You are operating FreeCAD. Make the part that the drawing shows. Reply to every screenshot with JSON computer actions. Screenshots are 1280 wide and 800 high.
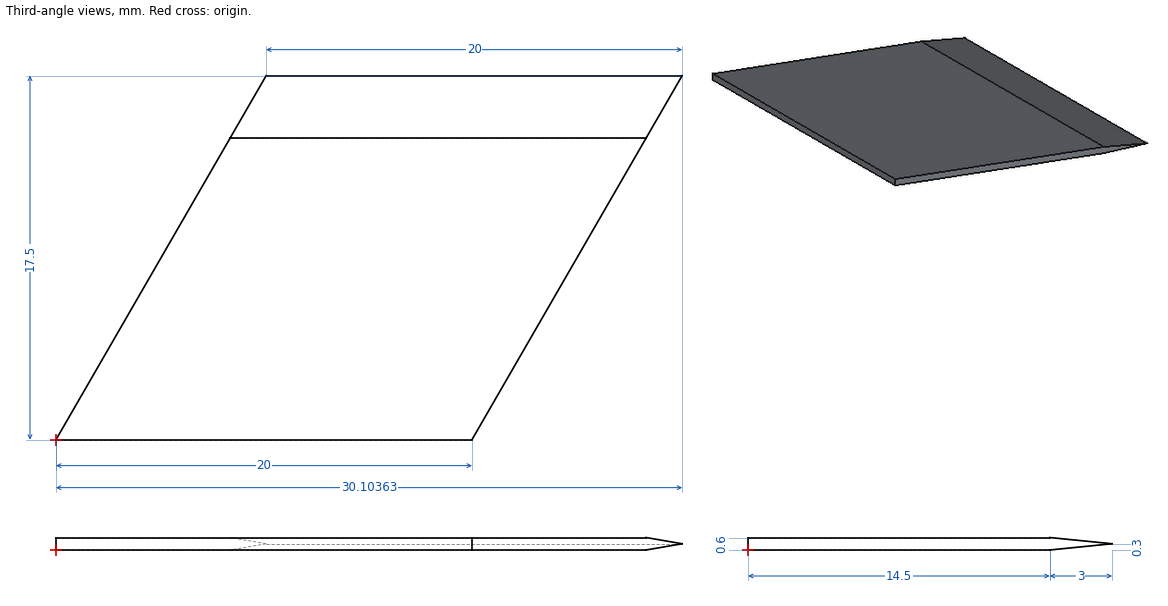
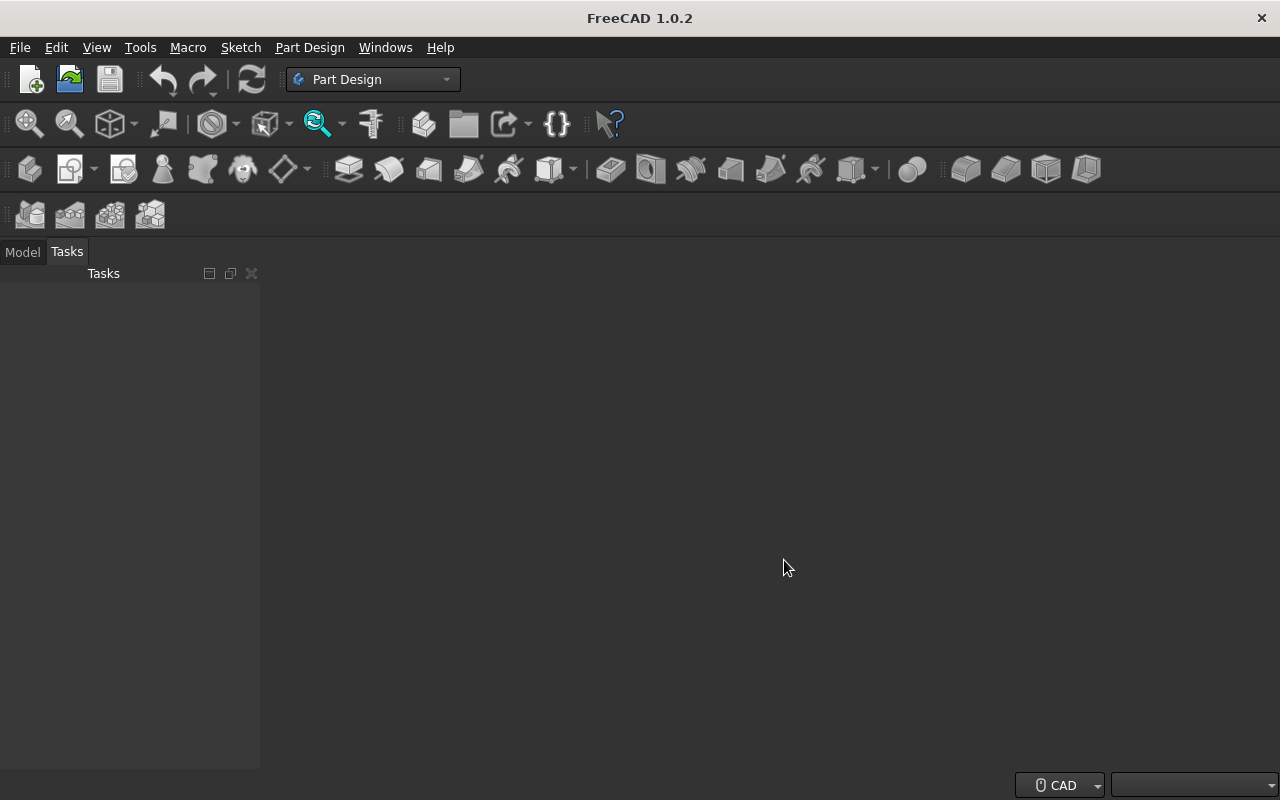
{"action": "left_click", "coordinate": [30, 80]}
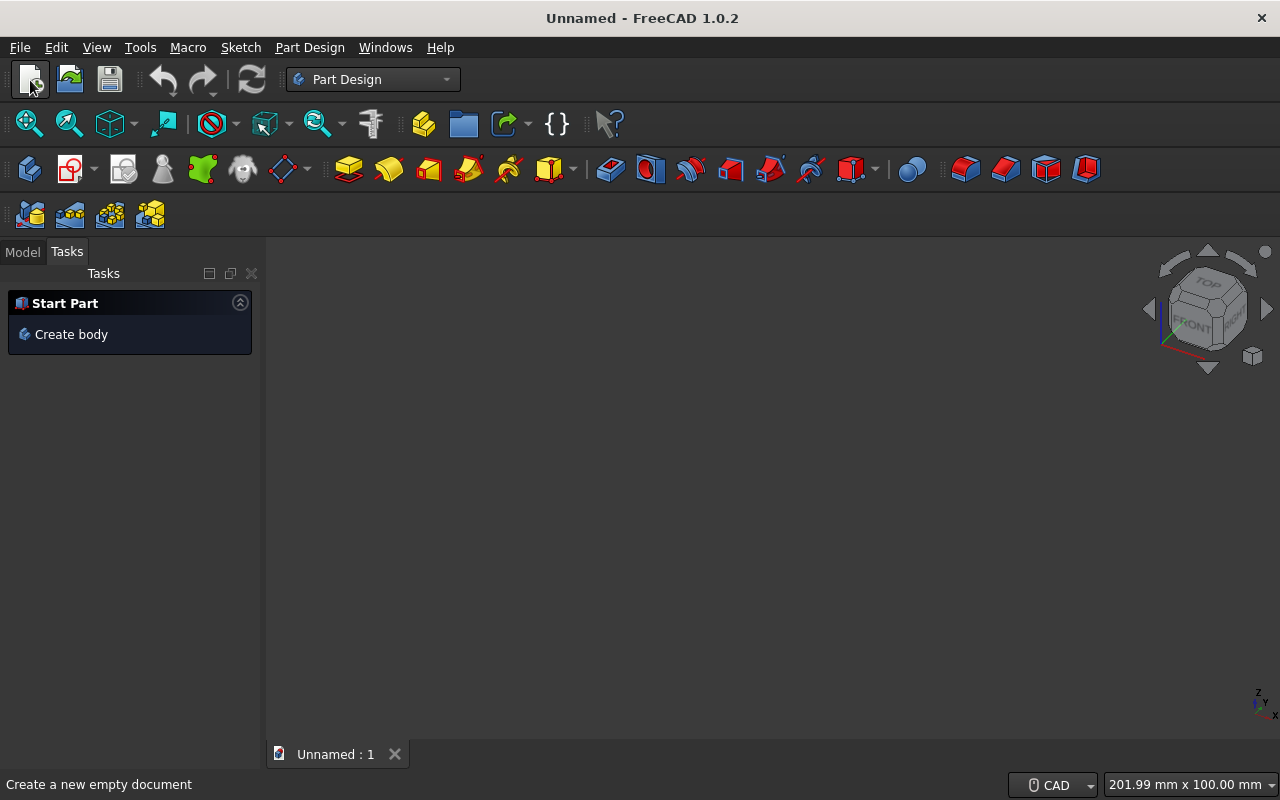
{"action": "left_click", "coordinate": [70, 170]}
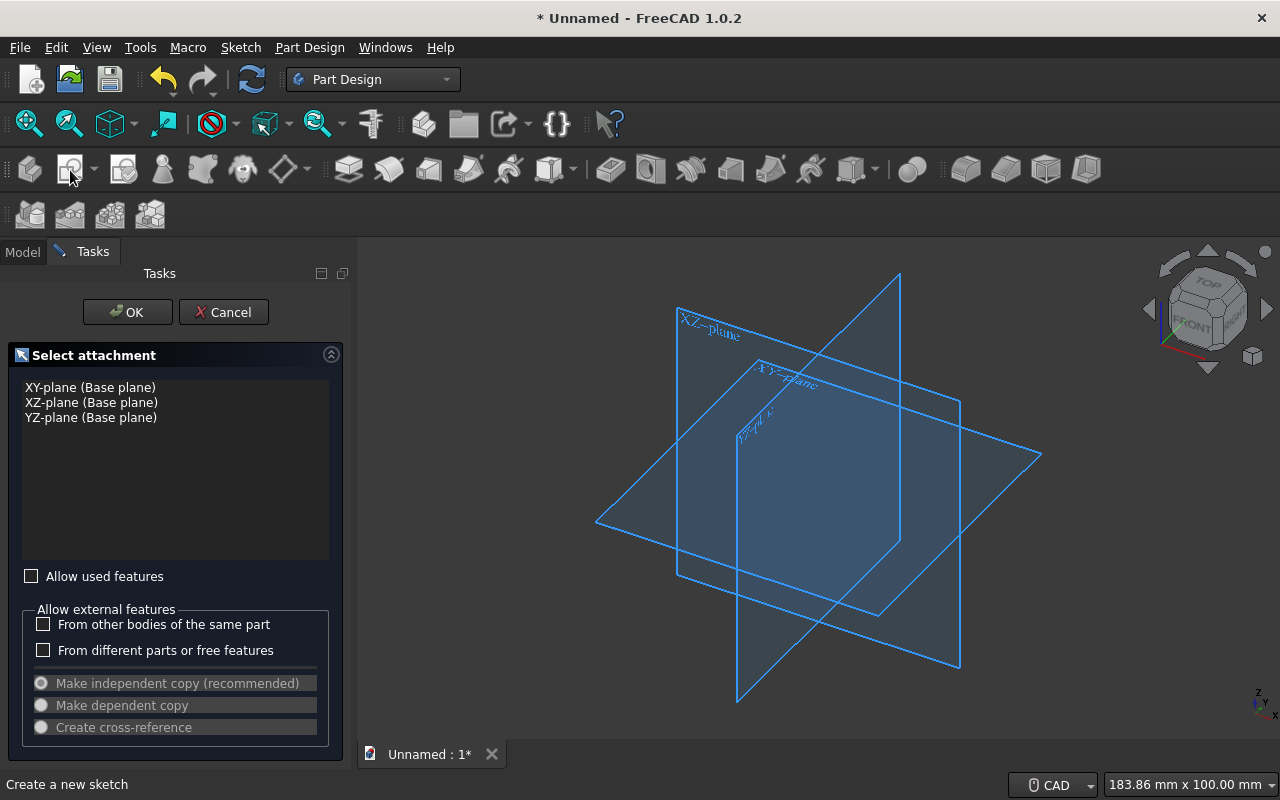
{"action": "left_click", "coordinate": [82, 388]}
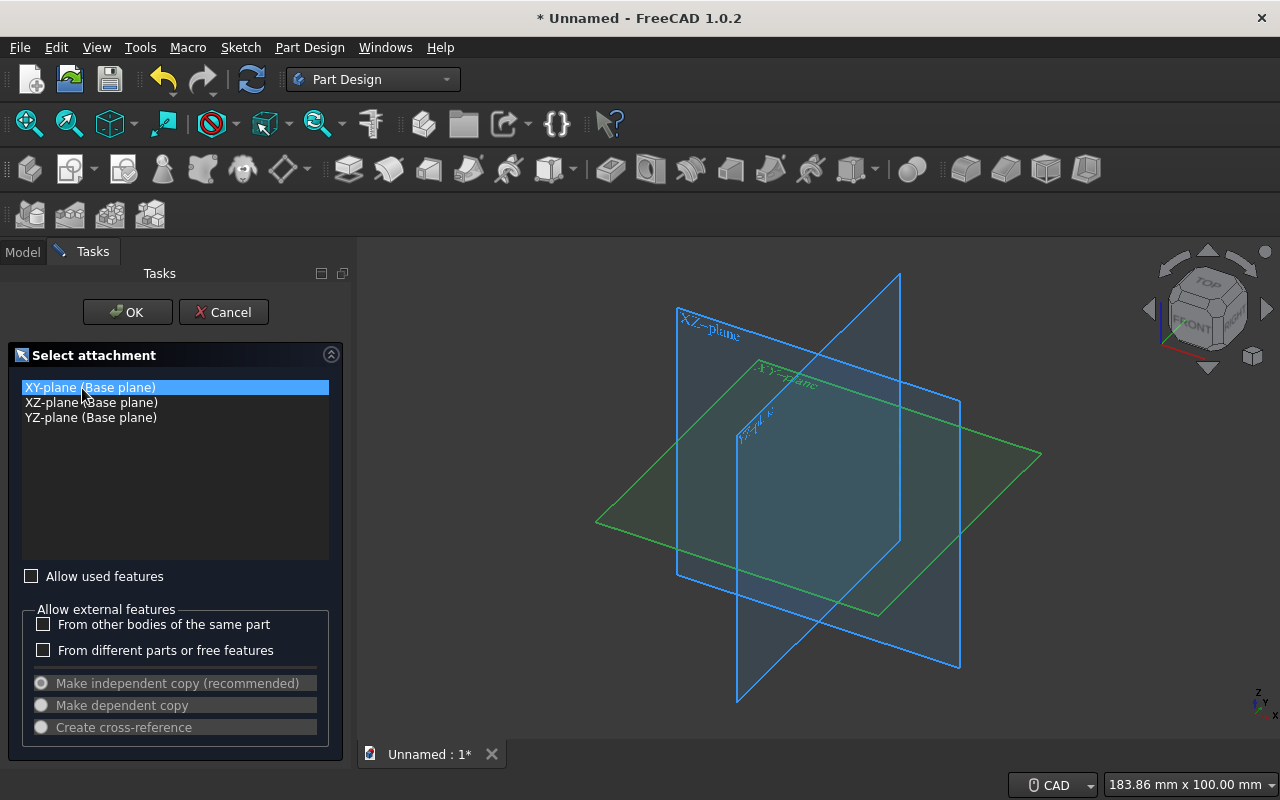
{"action": "left_click", "coordinate": [128, 312]}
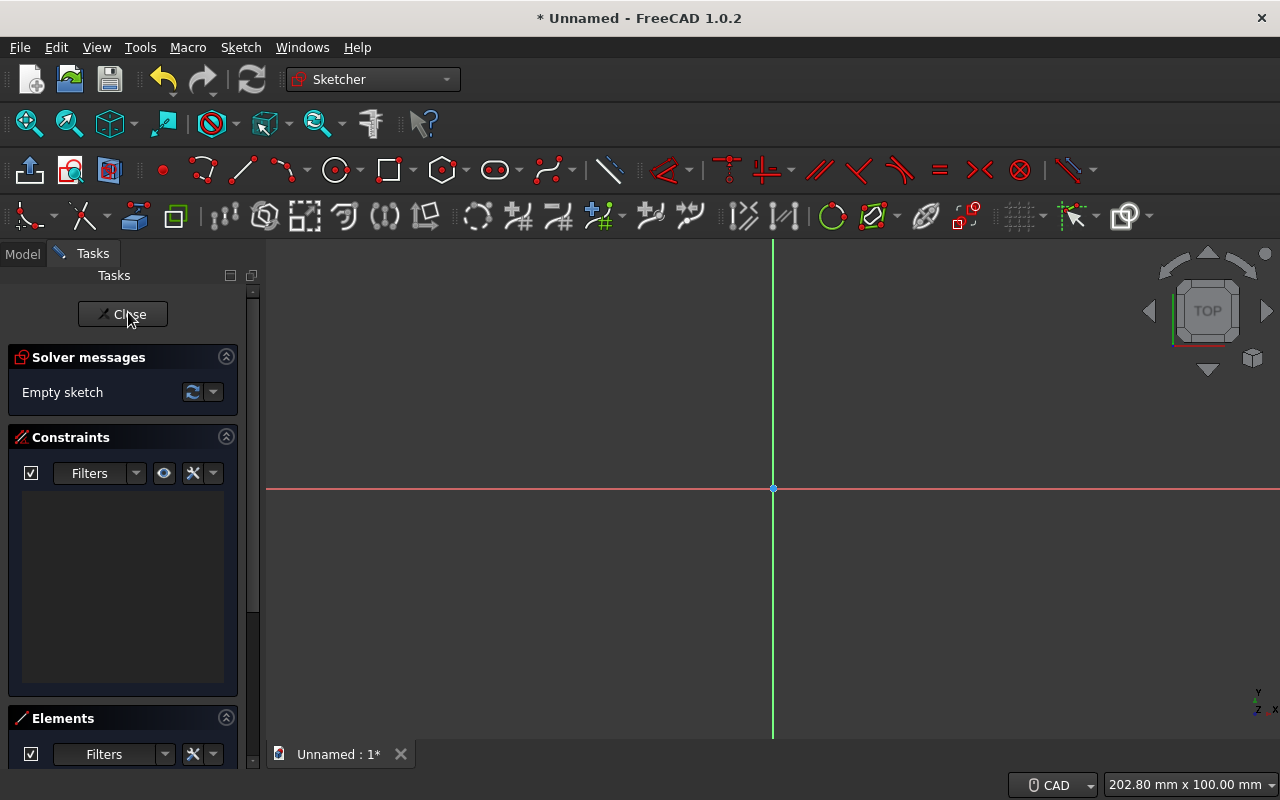
{"action": "scroll", "coordinate": [910, 426], "scroll_direction": "up", "scroll_amount": 6}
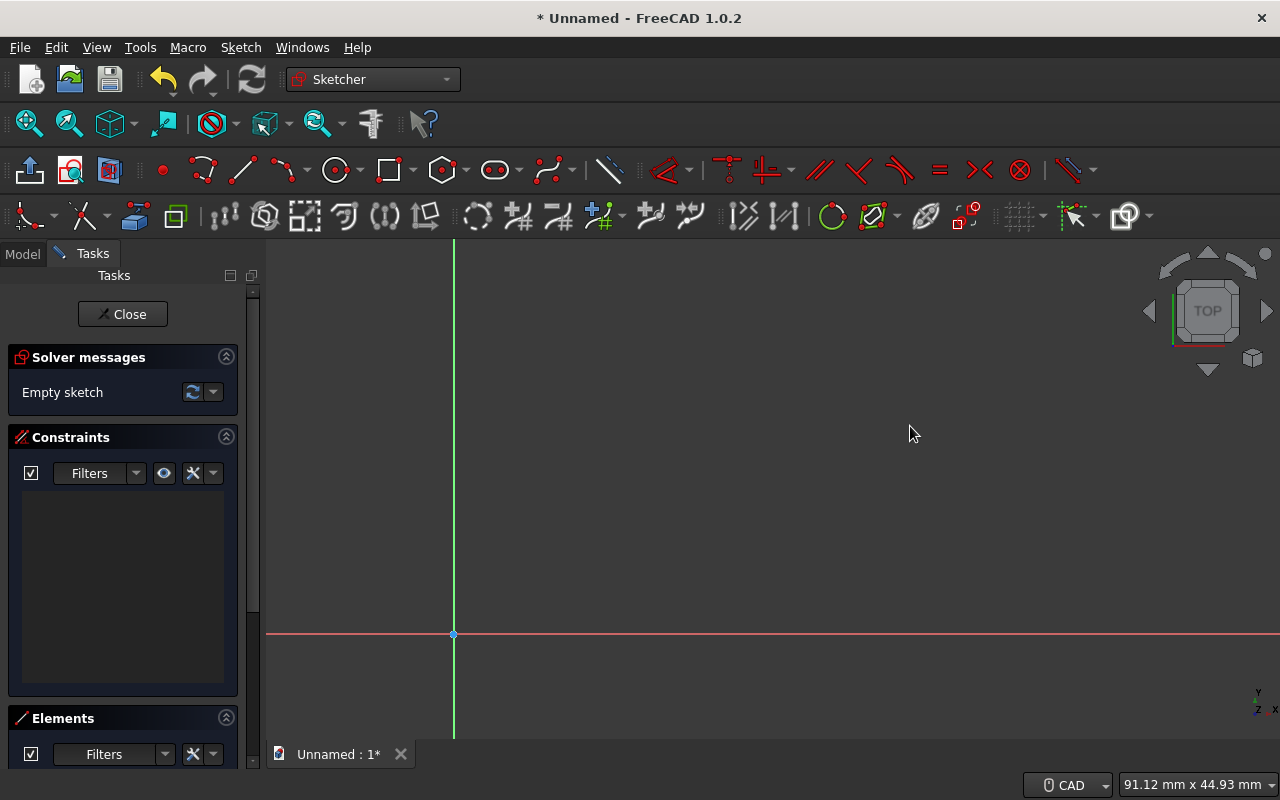
{"action": "left_click", "coordinate": [204, 170]}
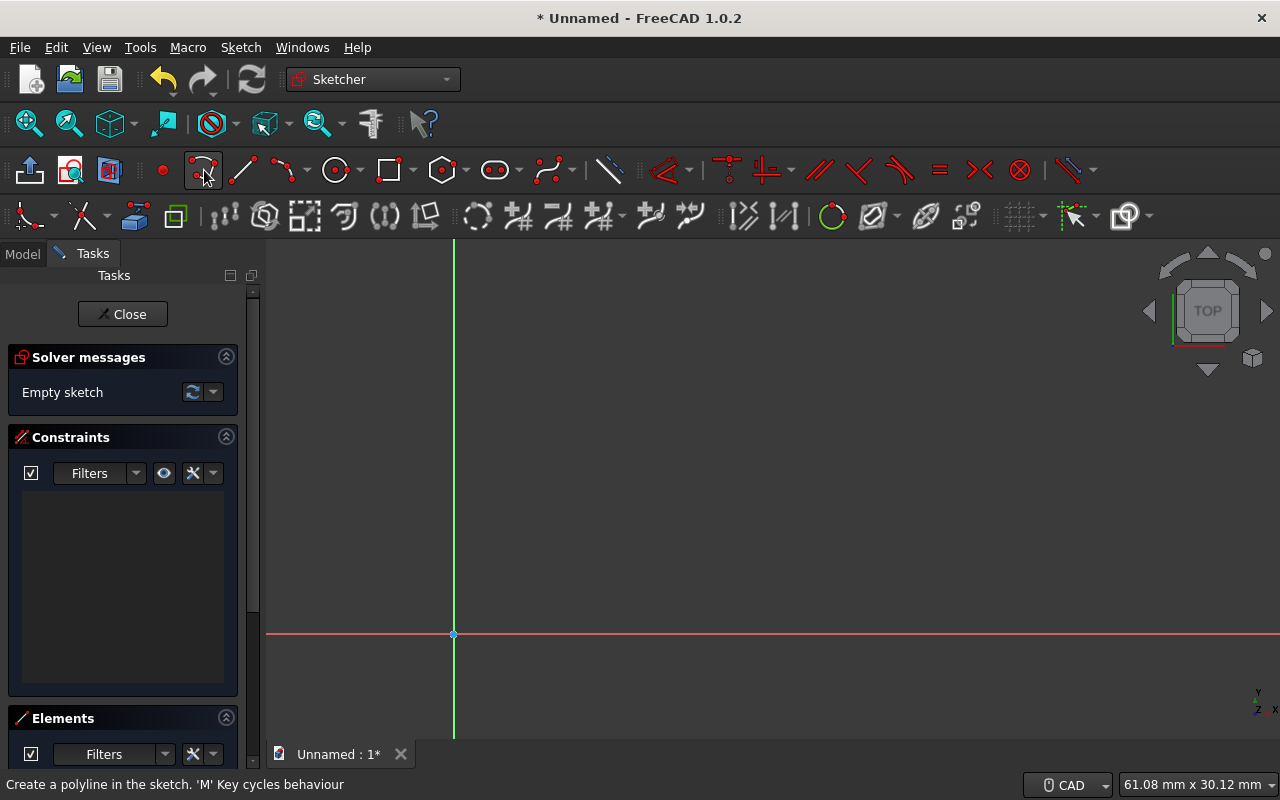
{"action": "left_click", "coordinate": [454, 634]}
{"action": "left_click", "coordinate": [786, 625]}
{"action": "left_click", "coordinate": [953, 344]}
{"action": "left_click", "coordinate": [621, 344]}
{"action": "left_click", "coordinate": [454, 634]}
{"action": "key", "text": "Escape"}
{"action": "key", "text": "Escape"}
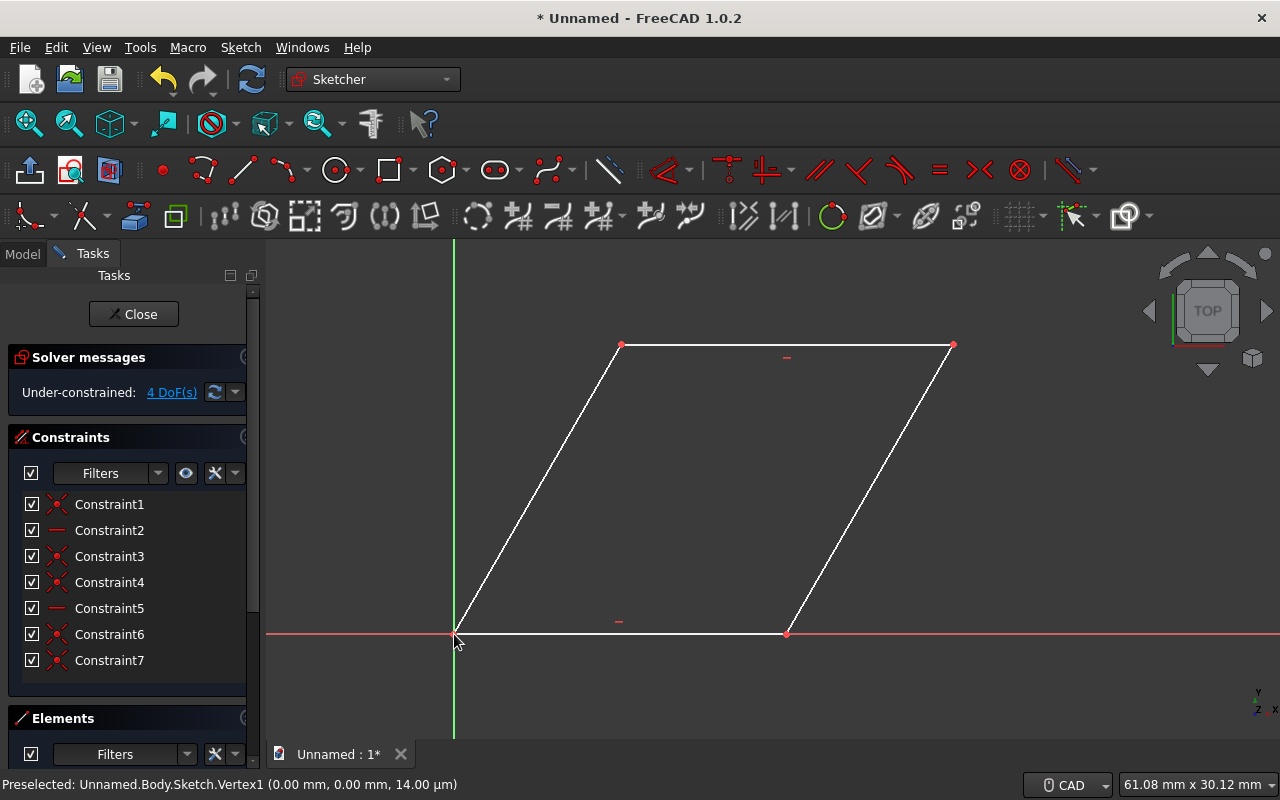
{"action": "left_click", "coordinate": [553, 634]}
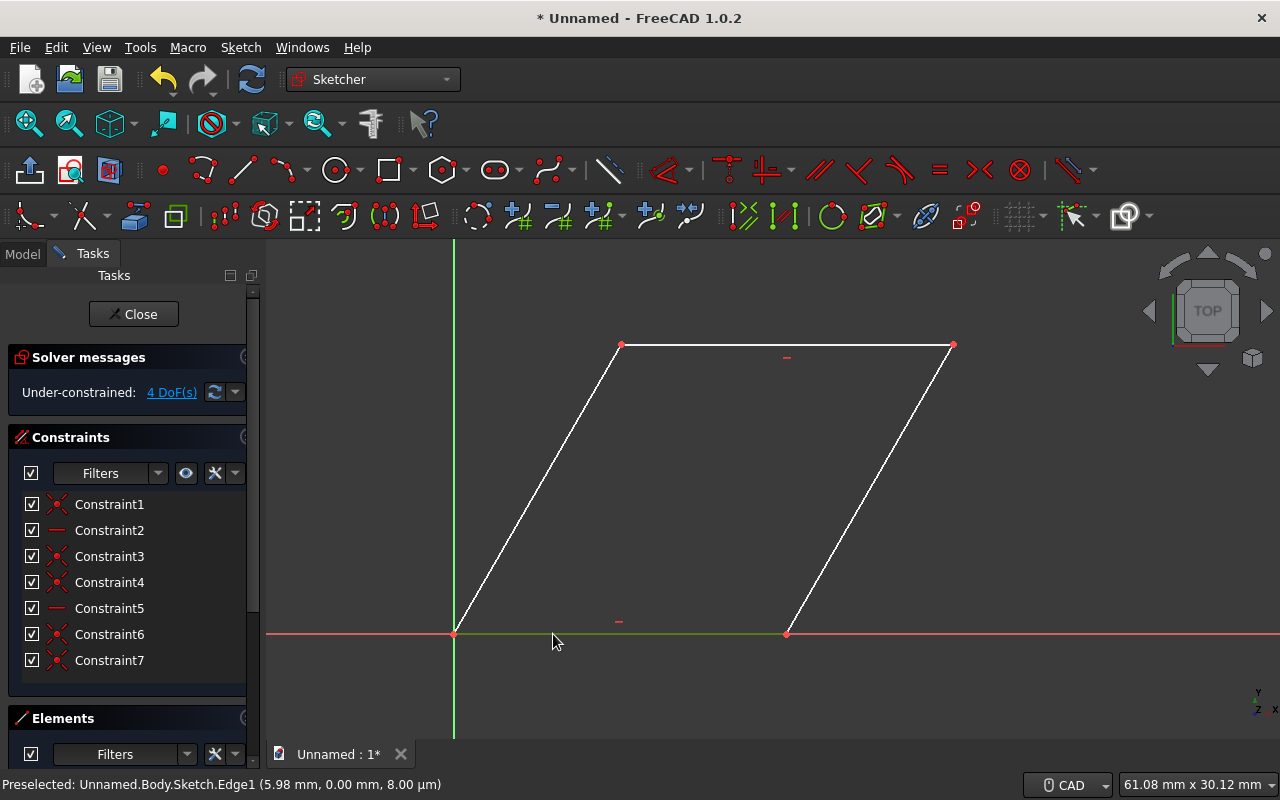
{"action": "left_click", "coordinate": [692, 170]}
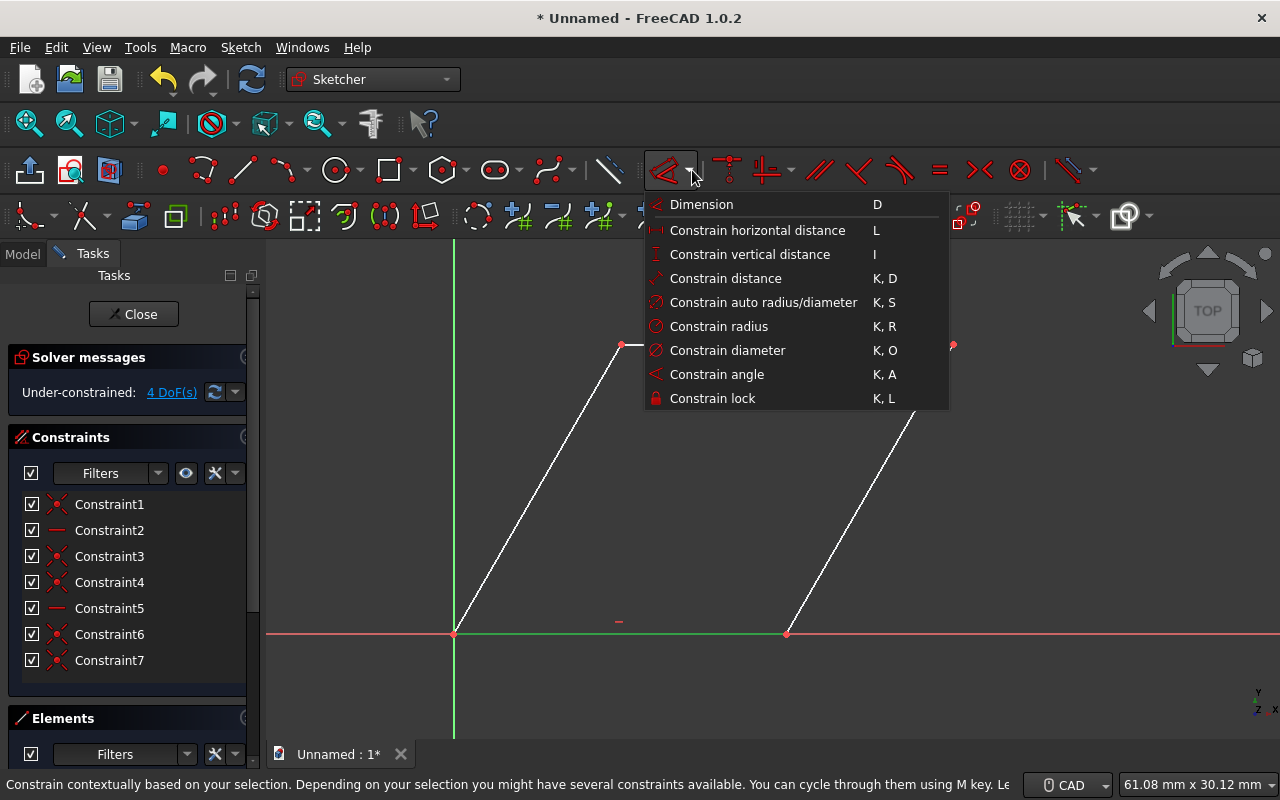
{"action": "left_click", "coordinate": [797, 230]}